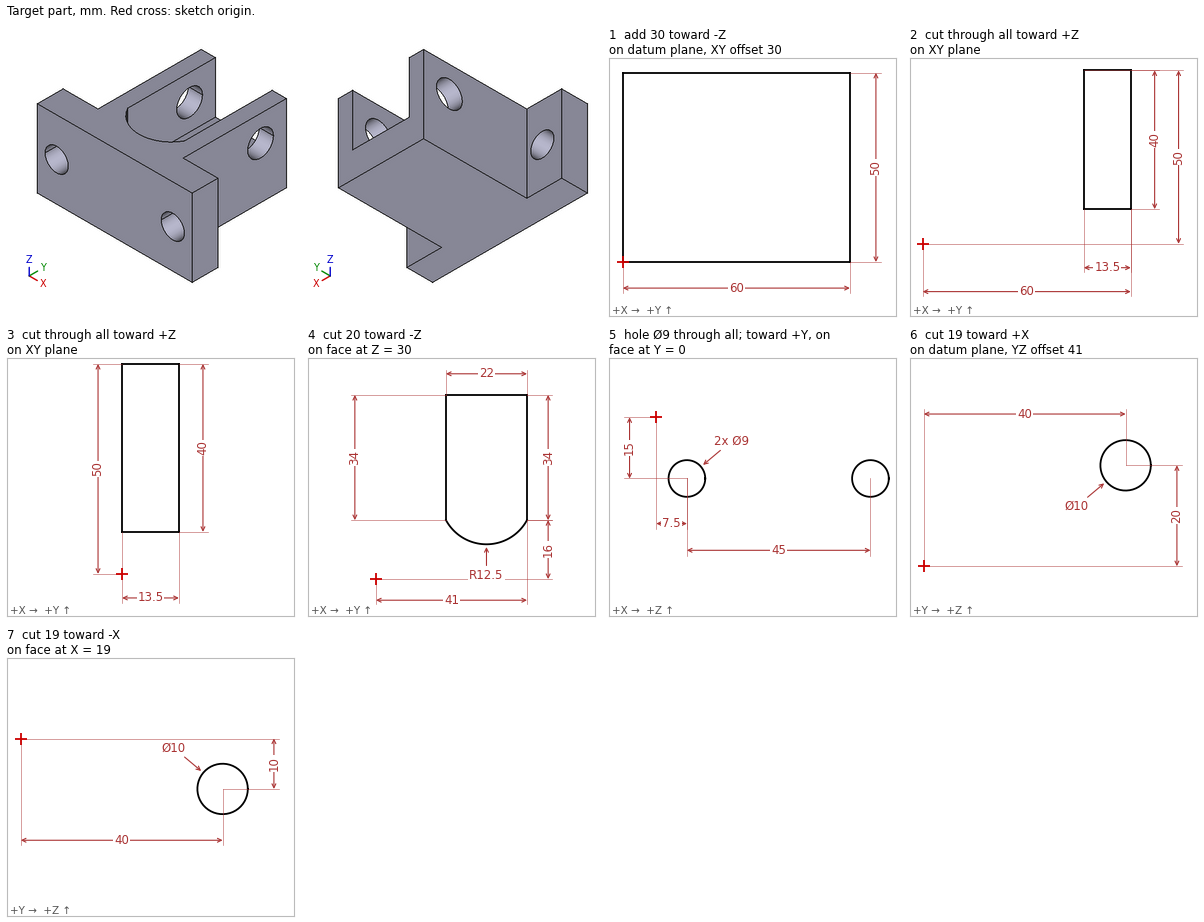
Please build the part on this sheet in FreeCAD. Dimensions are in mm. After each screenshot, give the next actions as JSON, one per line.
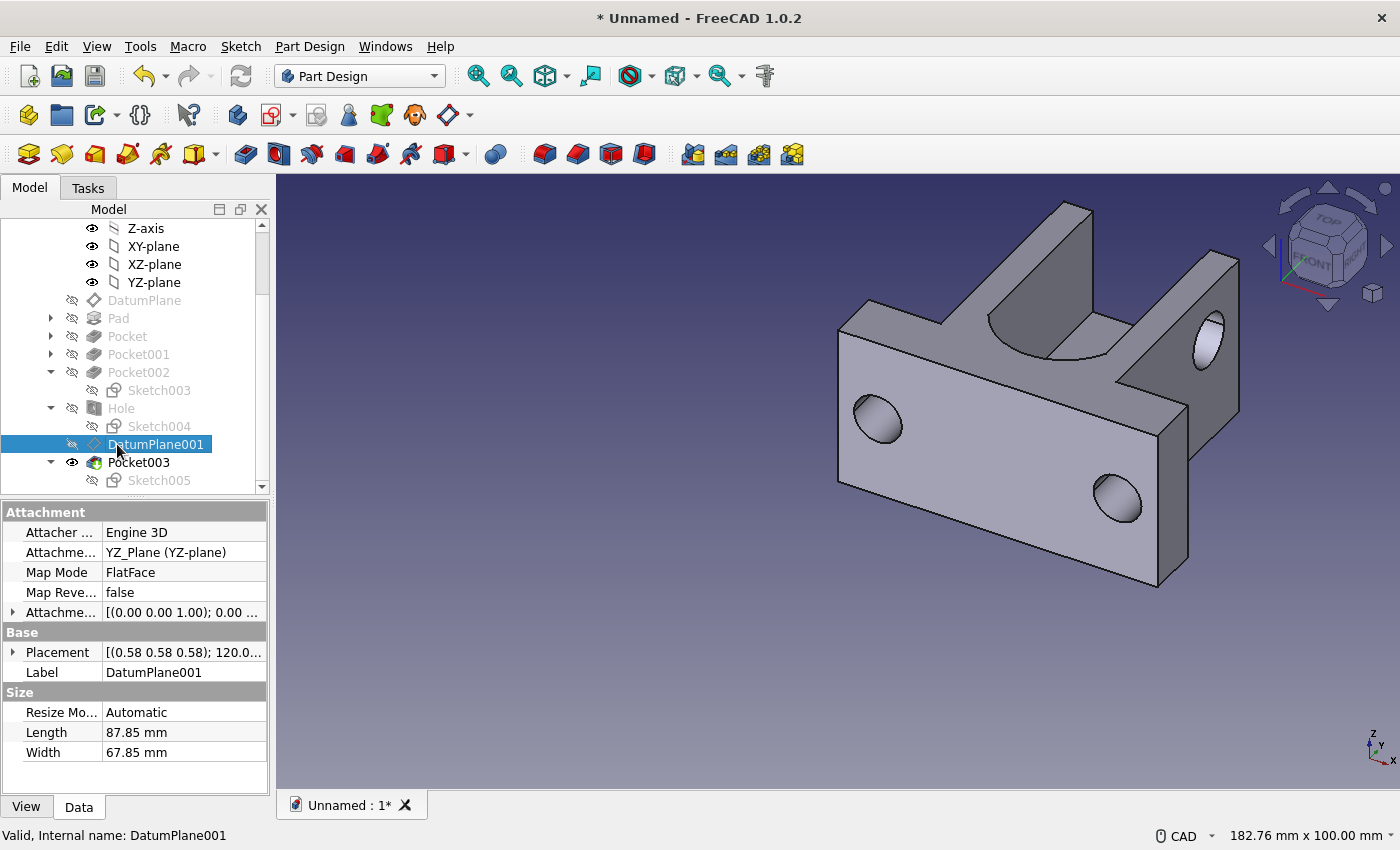
{"action": "left_click", "coordinate": [1056, 298]}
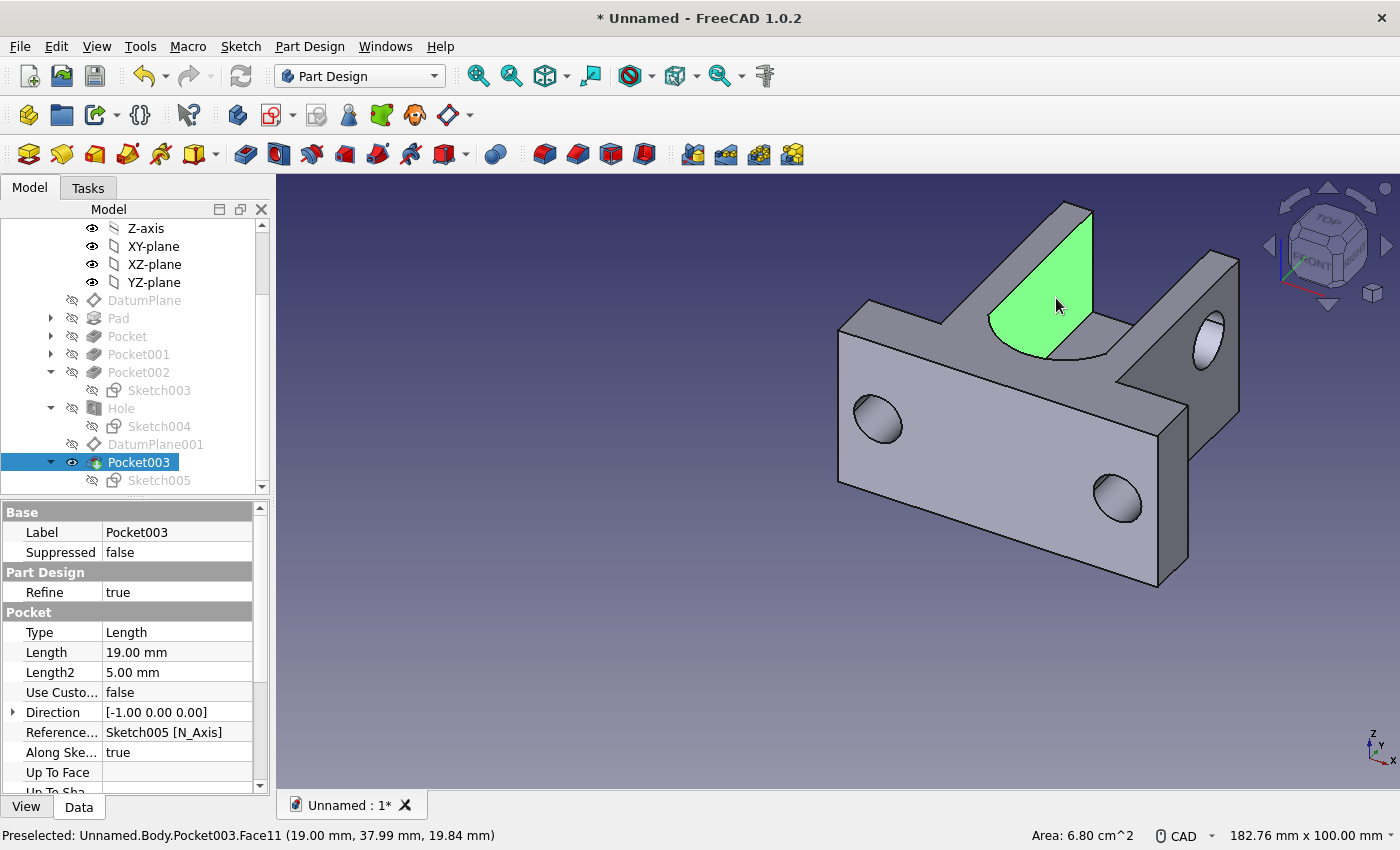
{"action": "left_click", "coordinate": [270, 116]}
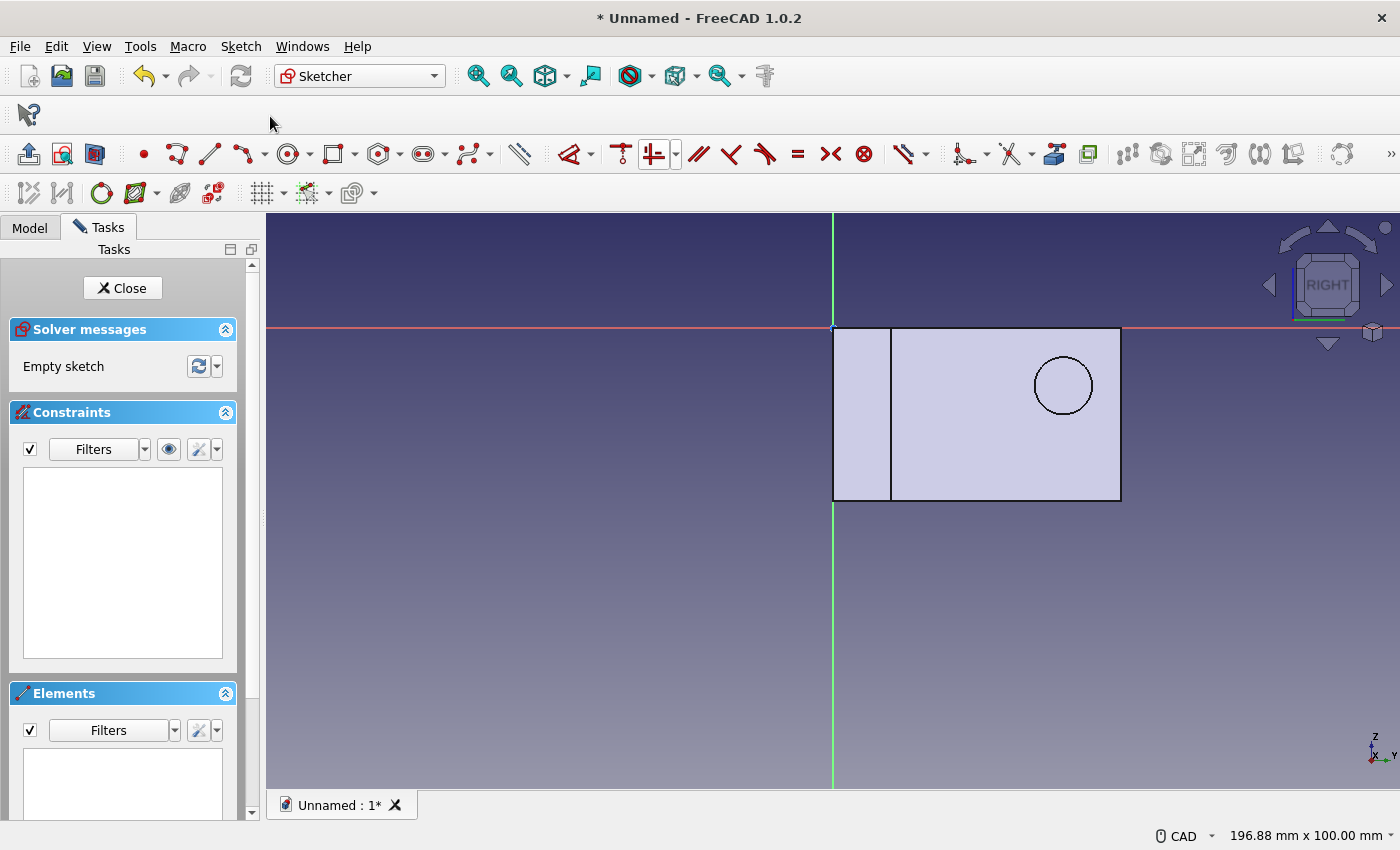
{"action": "scroll", "coordinate": [1123, 363], "scroll_direction": "up", "scroll_amount": 9}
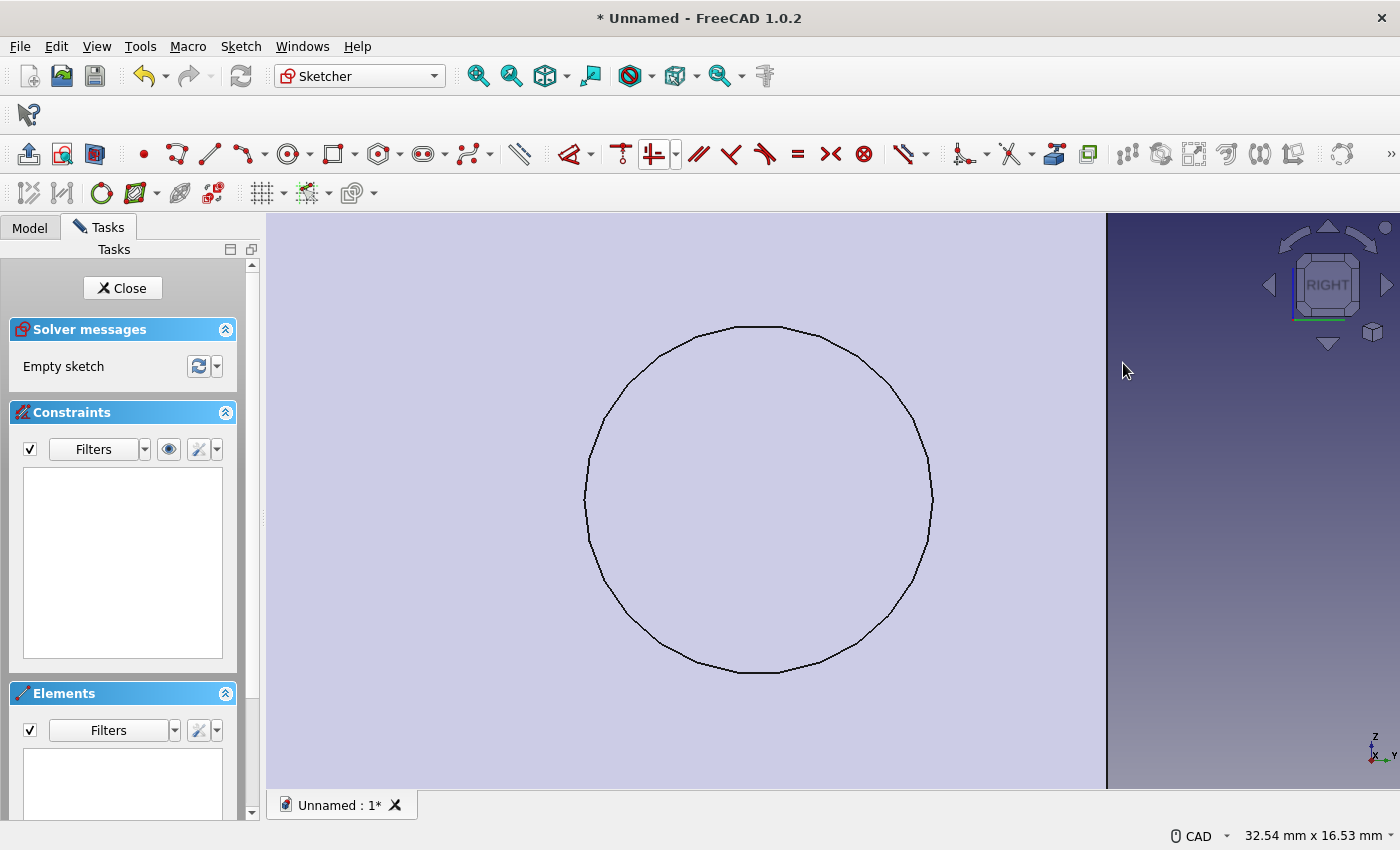
{"action": "left_click", "coordinate": [288, 154]}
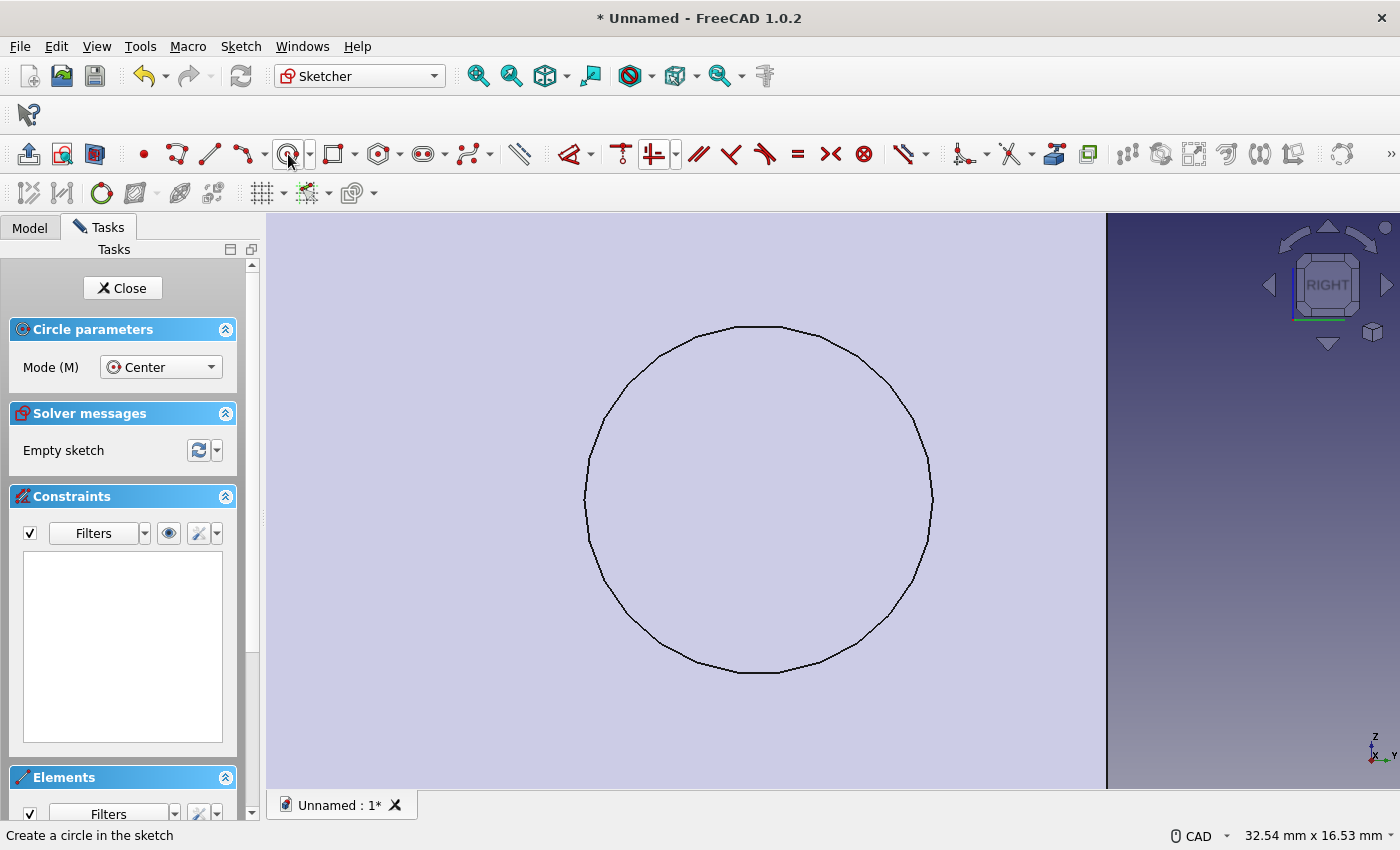
{"action": "left_click", "coordinate": [759, 500]}
{"action": "mouse_move", "coordinate": [882, 376]}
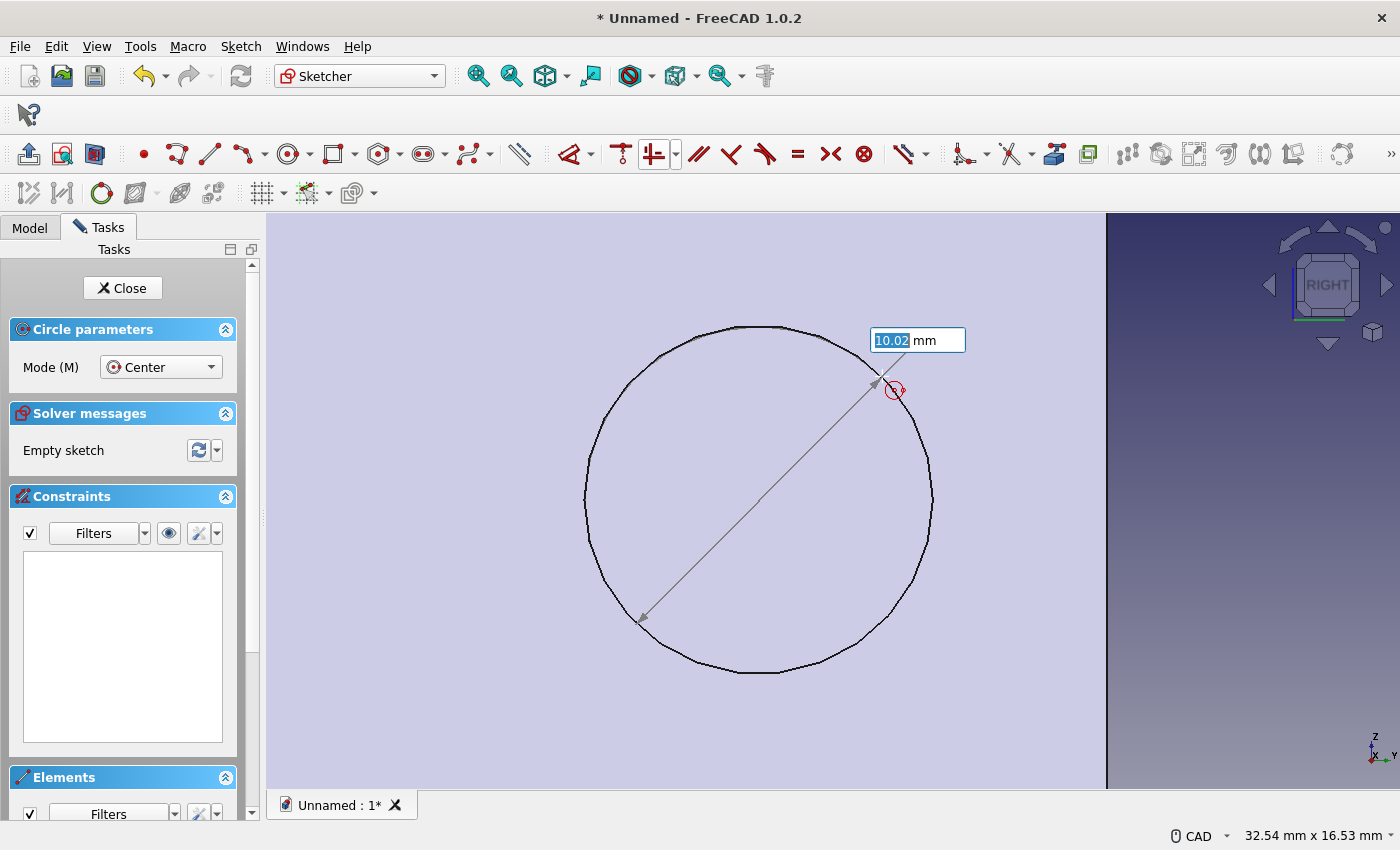
{"action": "type", "text": "10"}
{"action": "key", "text": "Return"}
{"action": "key", "text": "Escape"}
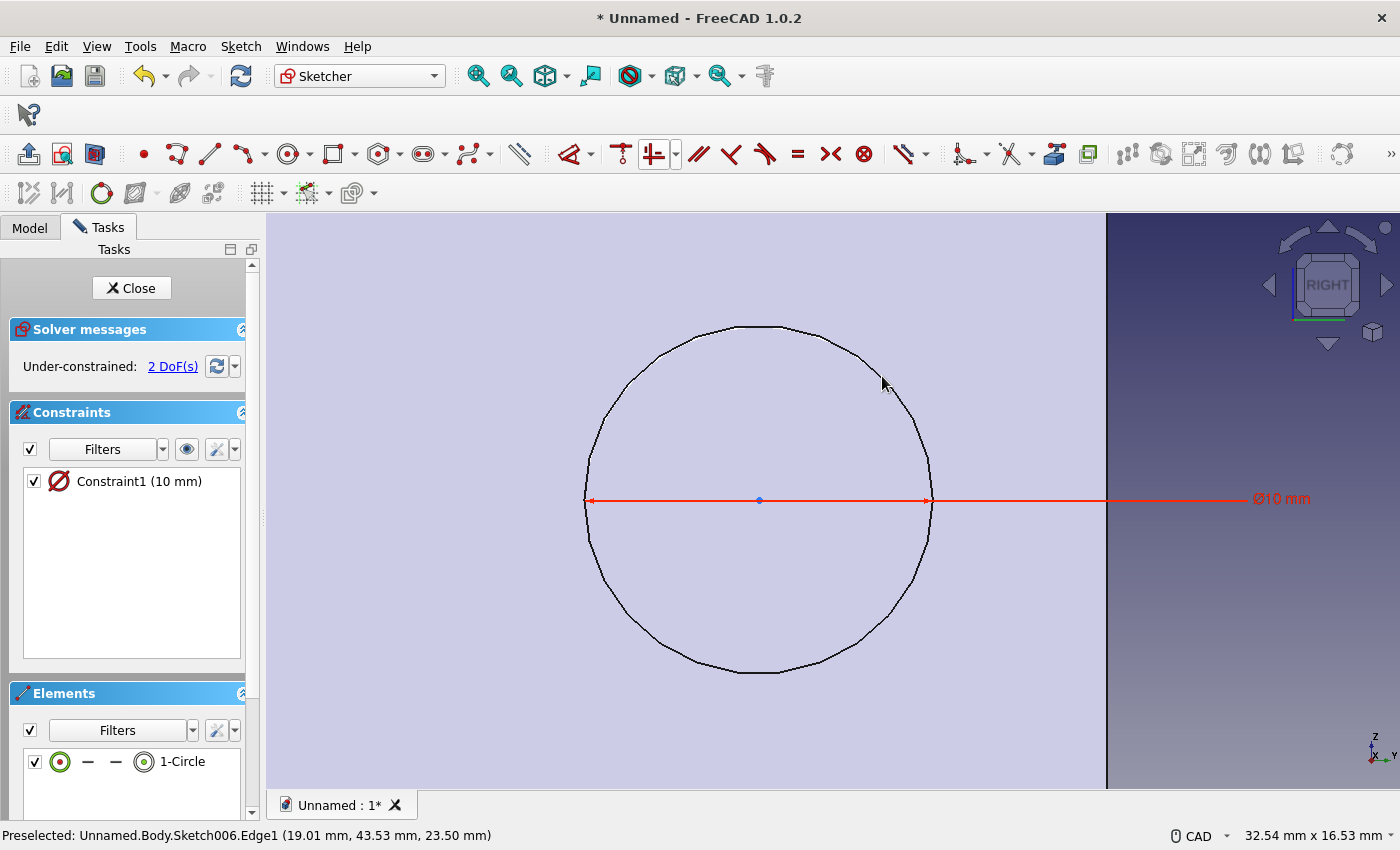
{"action": "left_click", "coordinate": [759, 501]}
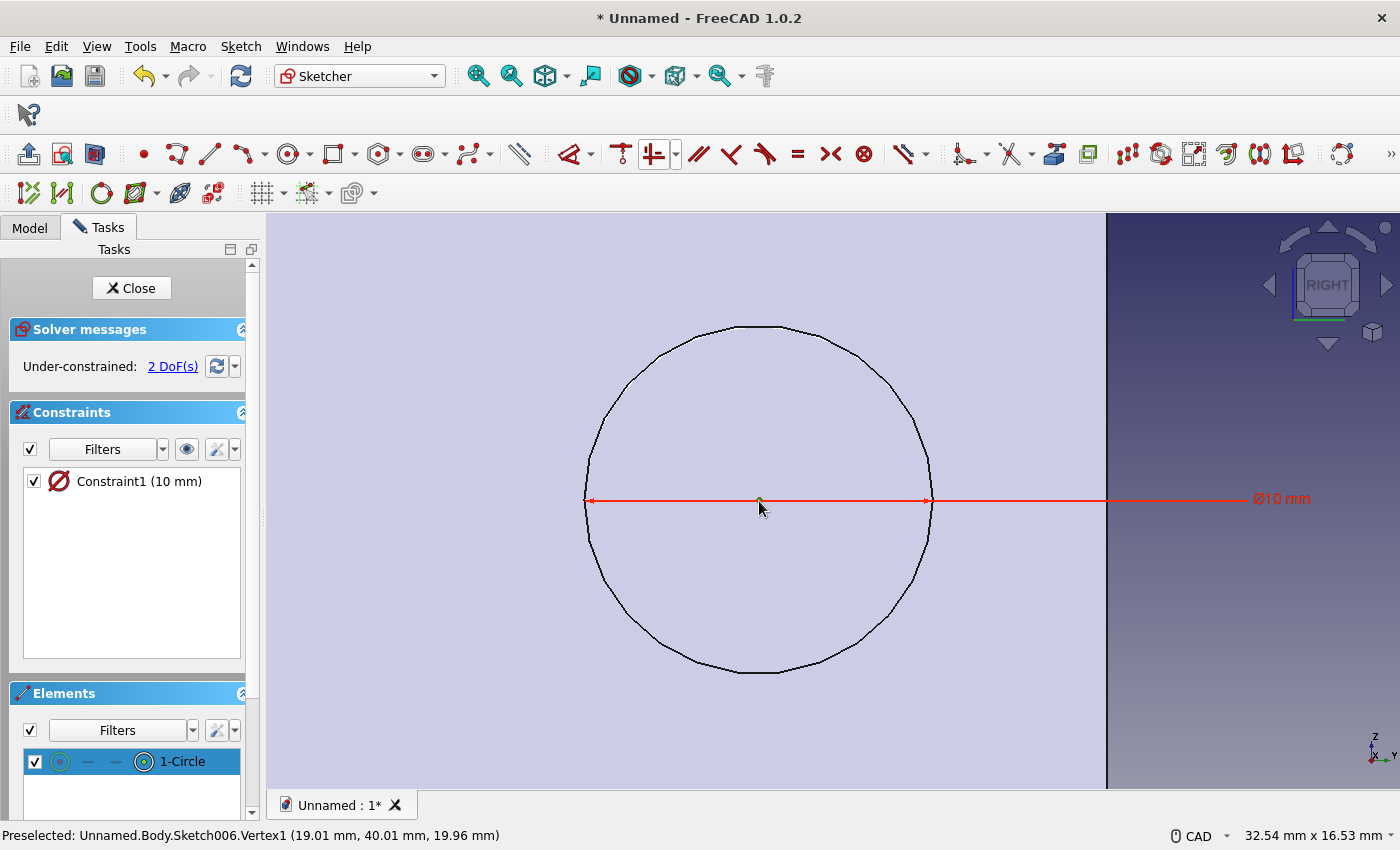
{"action": "key", "text": "l"}